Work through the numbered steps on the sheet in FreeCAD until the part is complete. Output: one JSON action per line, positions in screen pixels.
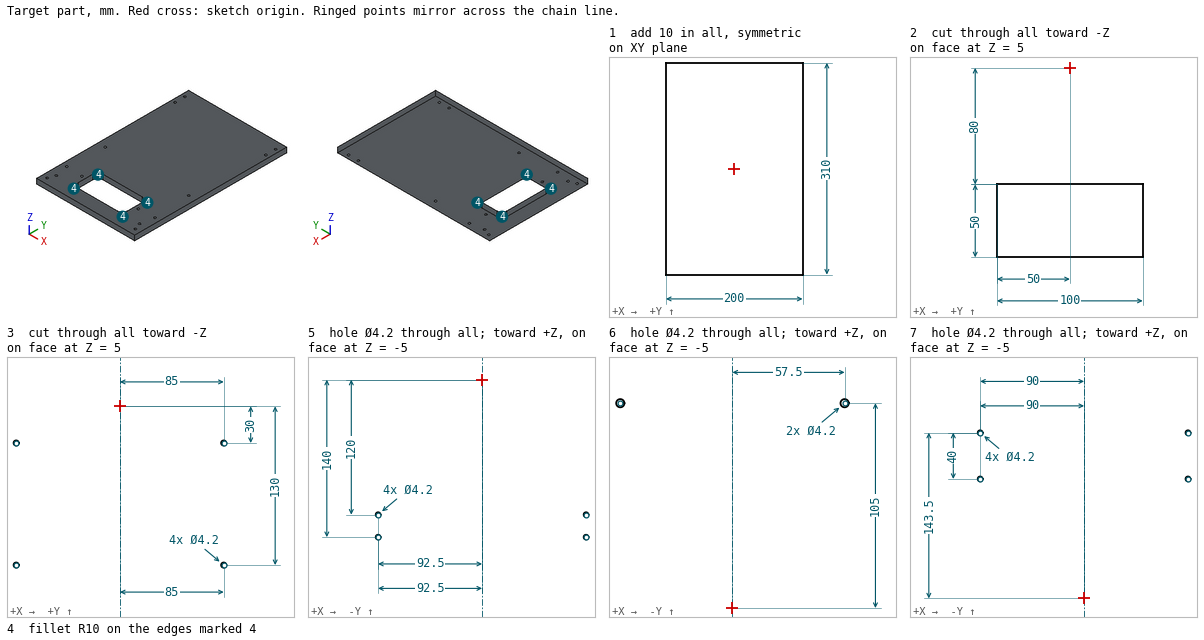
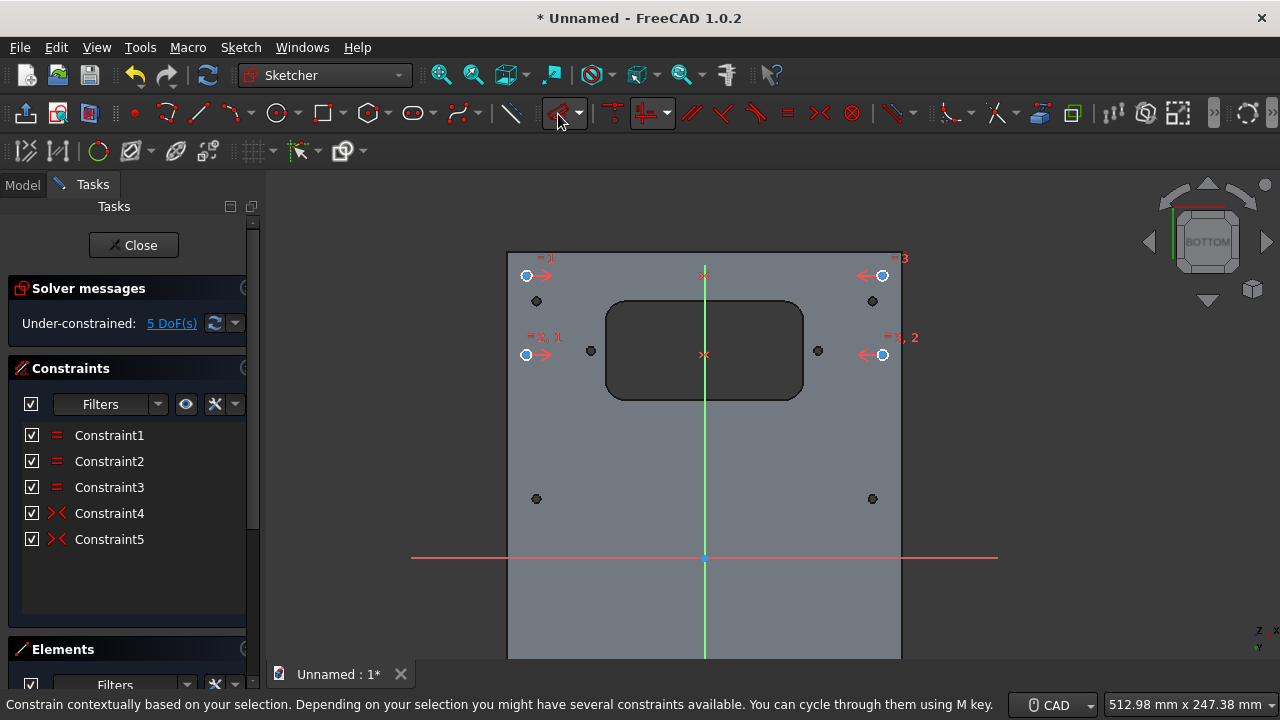
{"action": "scroll", "coordinate": [522, 276], "scroll_direction": "up", "scroll_amount": 8}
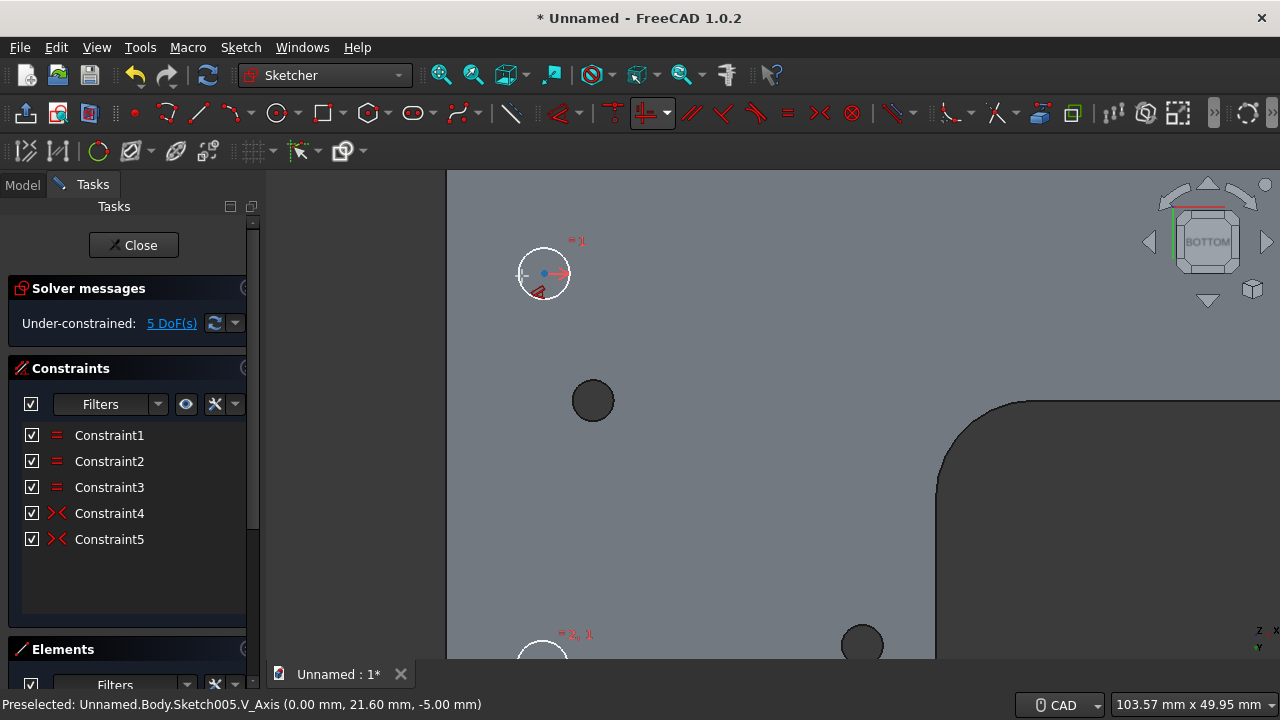
{"action": "left_click", "coordinate": [519, 273]}
{"action": "left_click", "coordinate": [487, 272]}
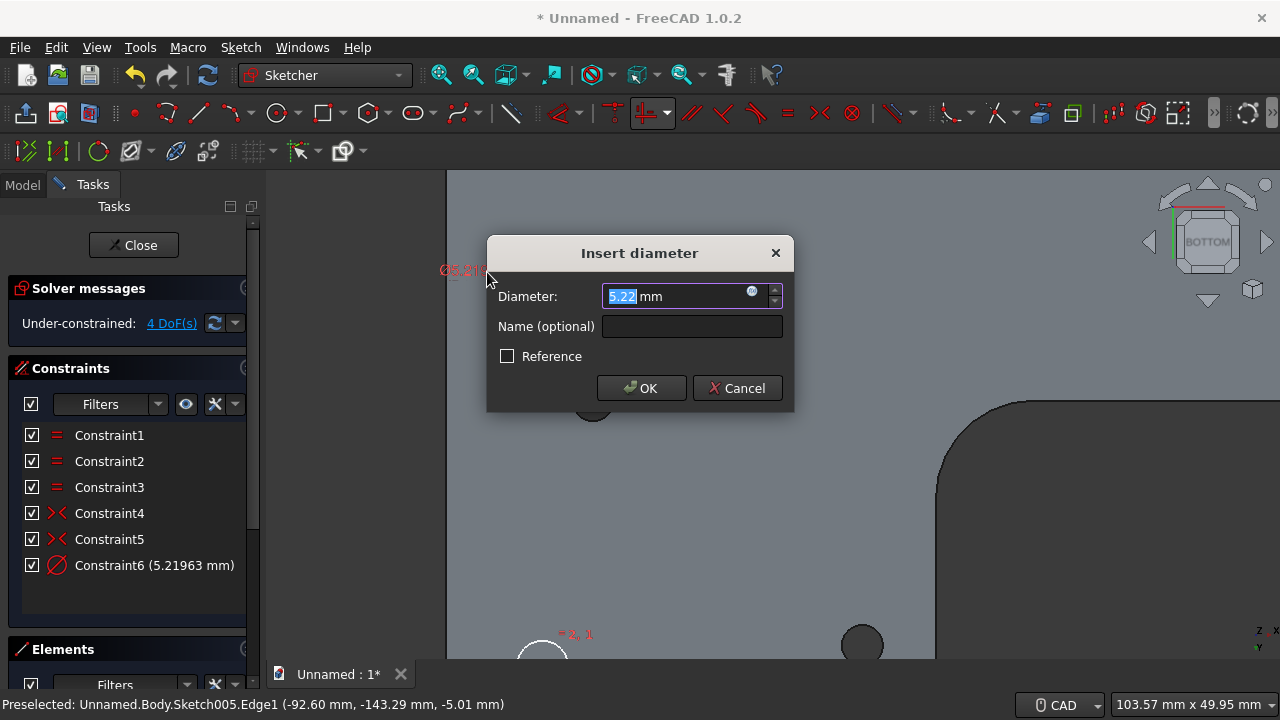
{"action": "type", "text": "4.2"}
{"action": "key", "text": "Return"}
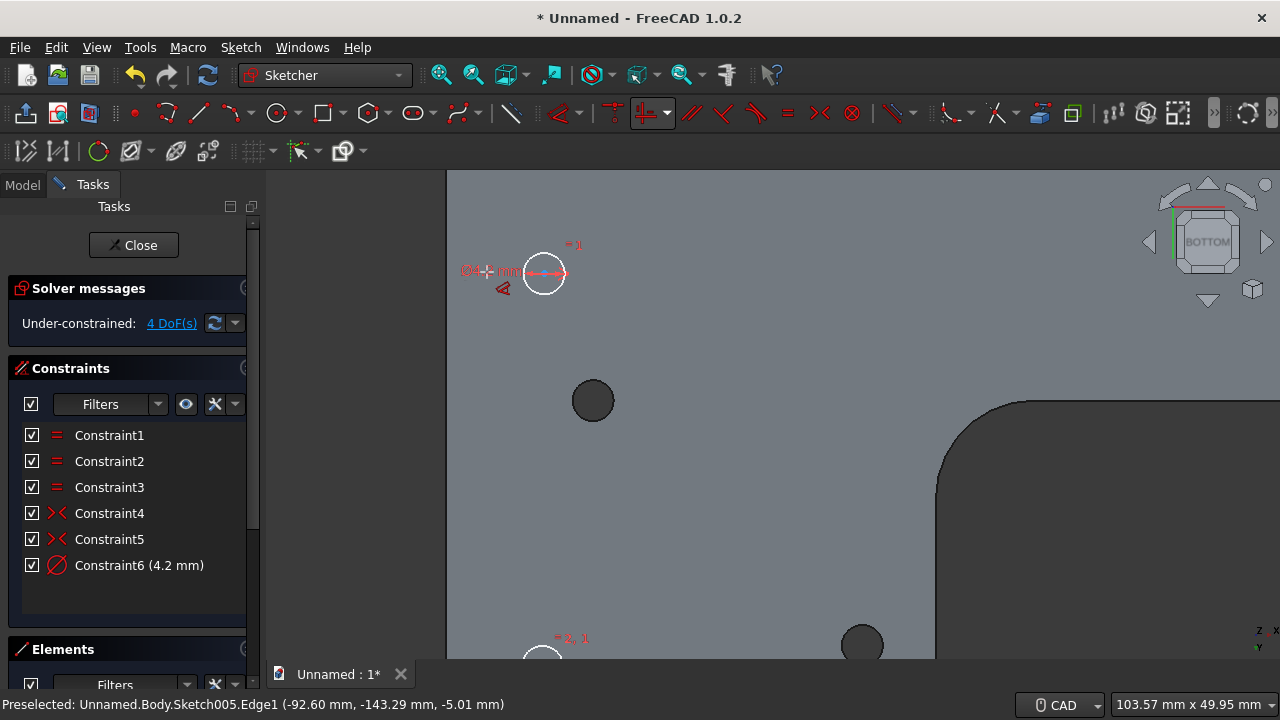
{"action": "scroll", "coordinate": [522, 276], "scroll_direction": "down", "scroll_amount": 8}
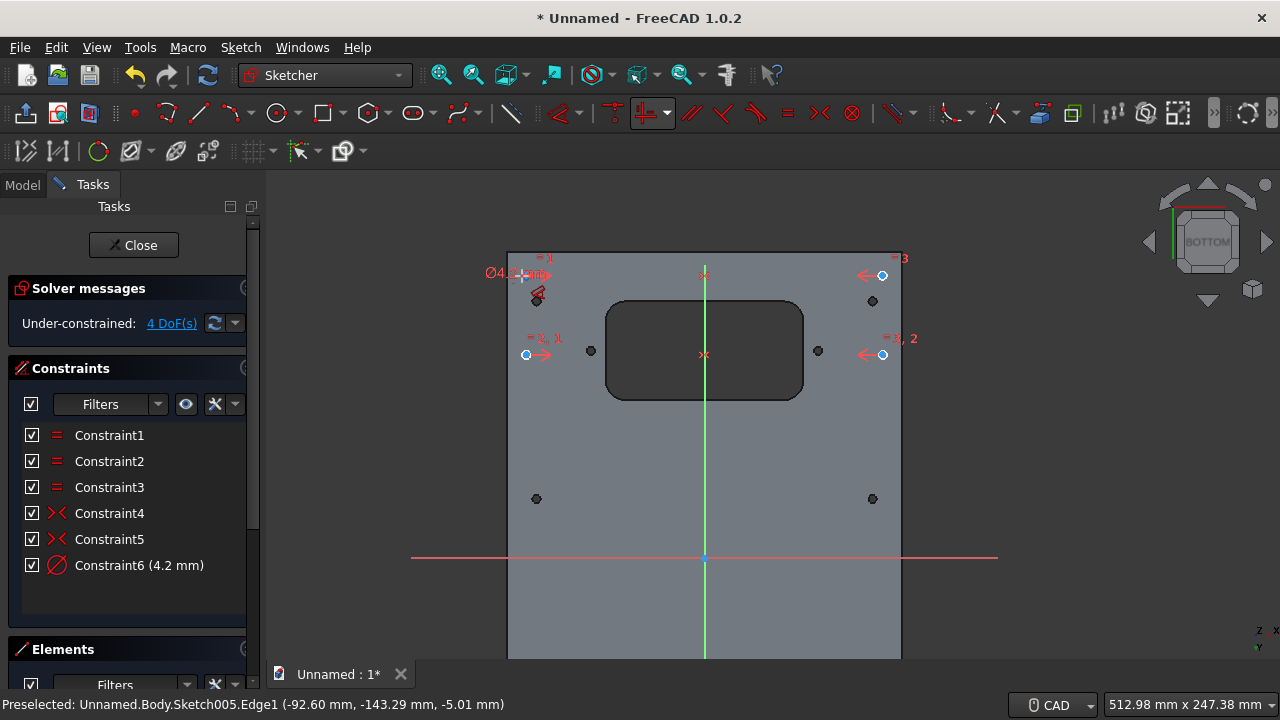
{"action": "left_click", "coordinate": [527, 276]}
{"action": "left_click", "coordinate": [616, 592]}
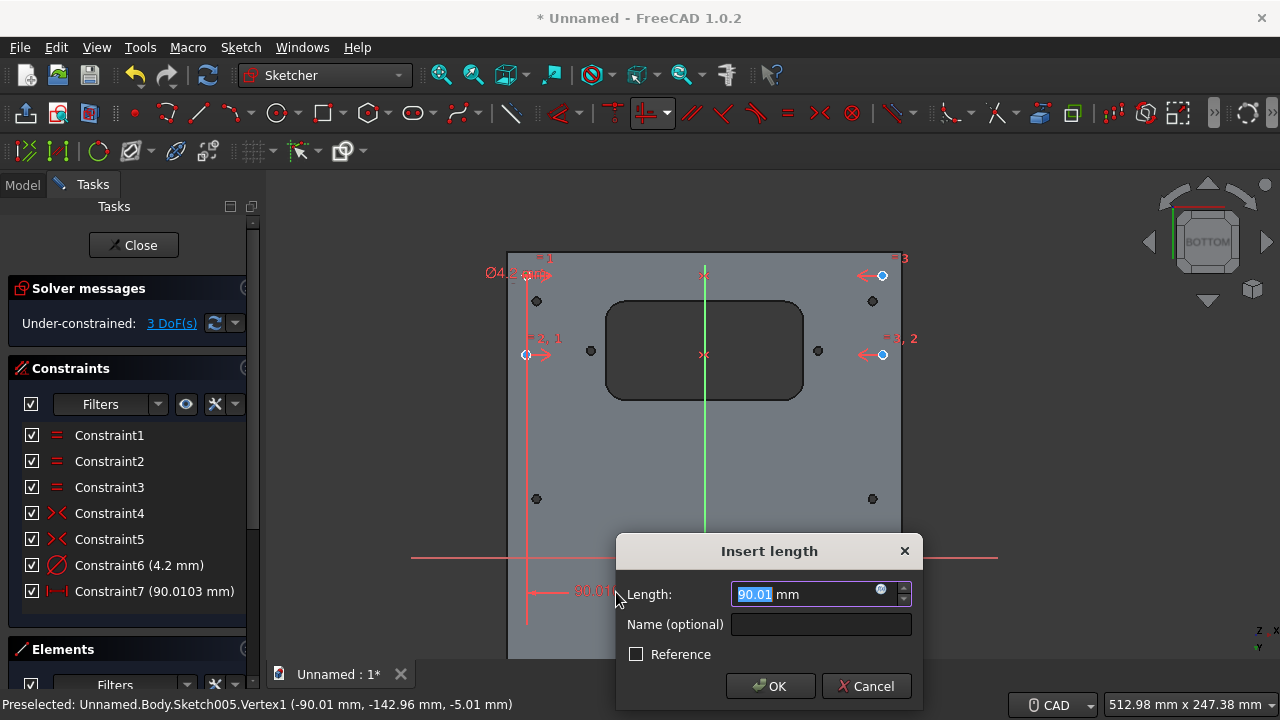
{"action": "type", "text": "90"}
{"action": "key", "text": "Return"}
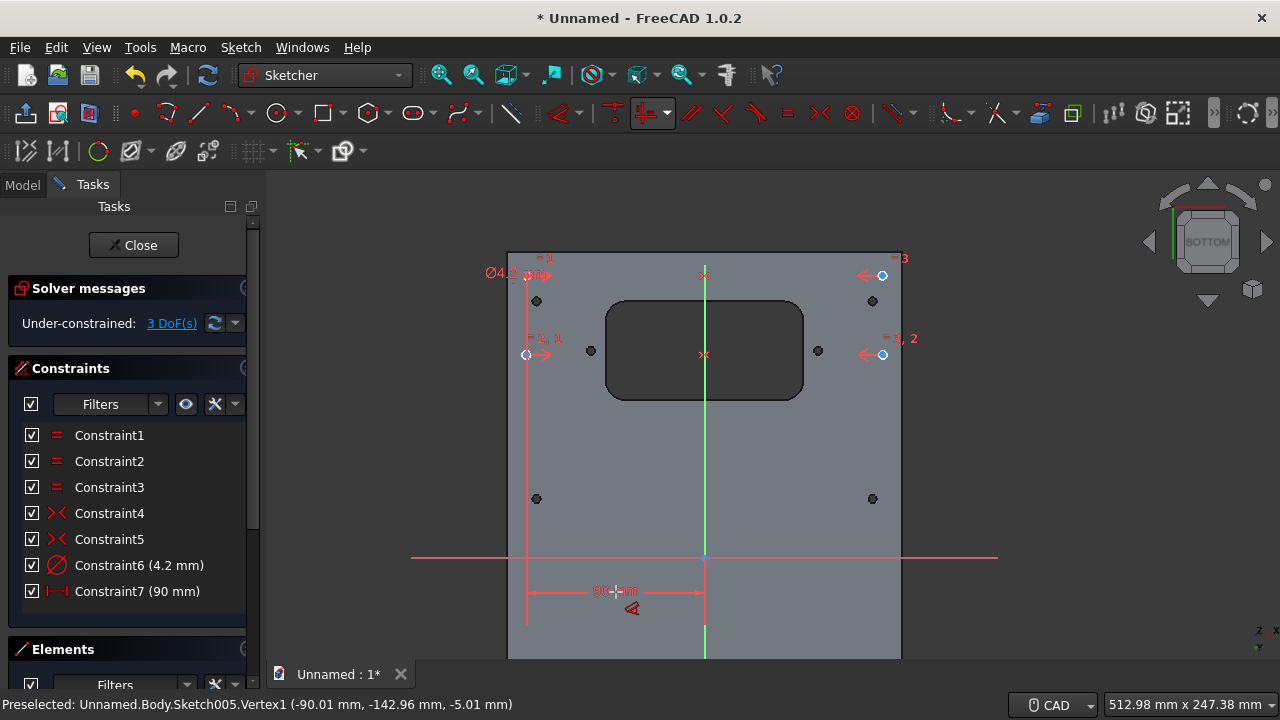
{"action": "left_click", "coordinate": [526, 355]}
{"action": "left_click", "coordinate": [615, 321]}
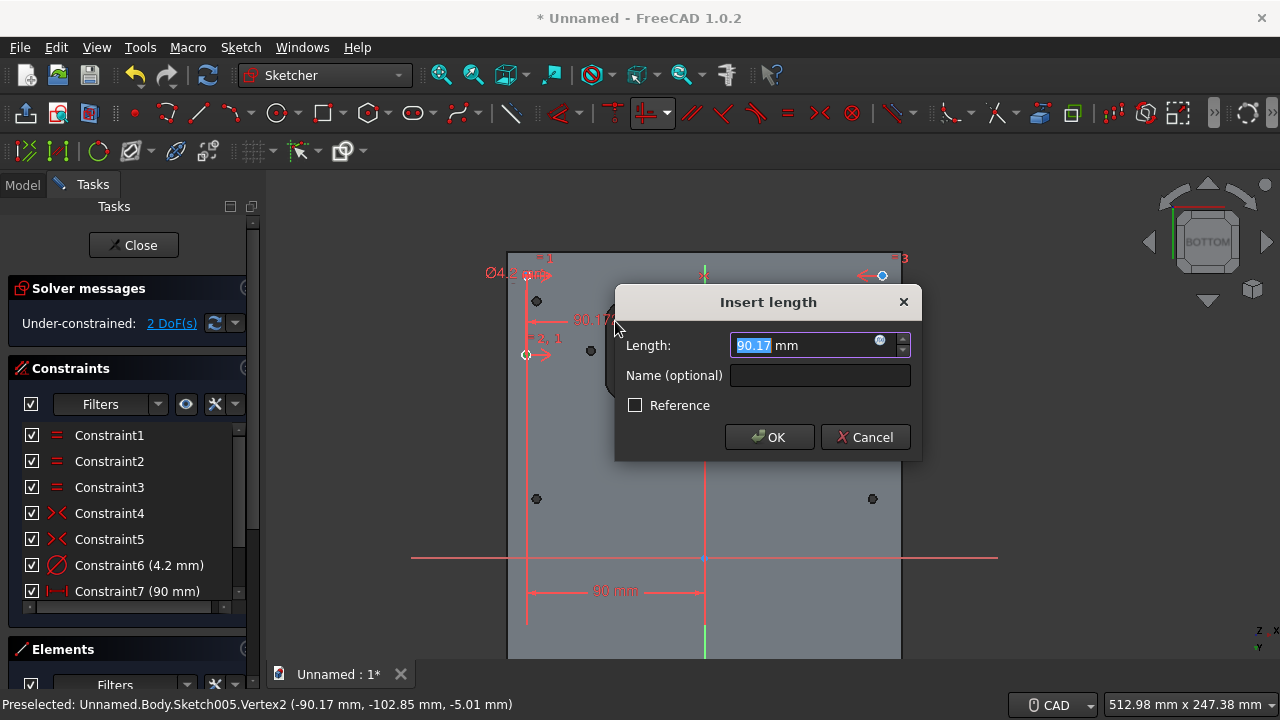
{"action": "type", "text": "90"}
{"action": "key", "text": "Return"}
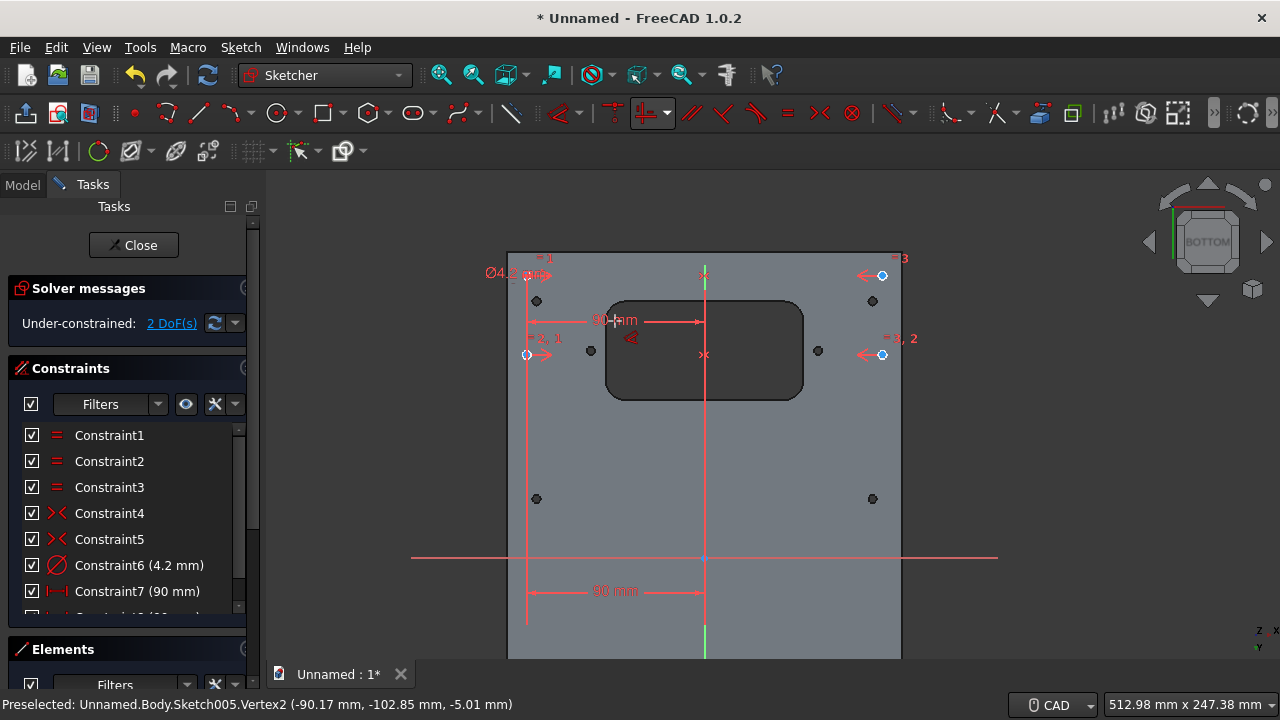
{"action": "left_click", "coordinate": [527, 276]}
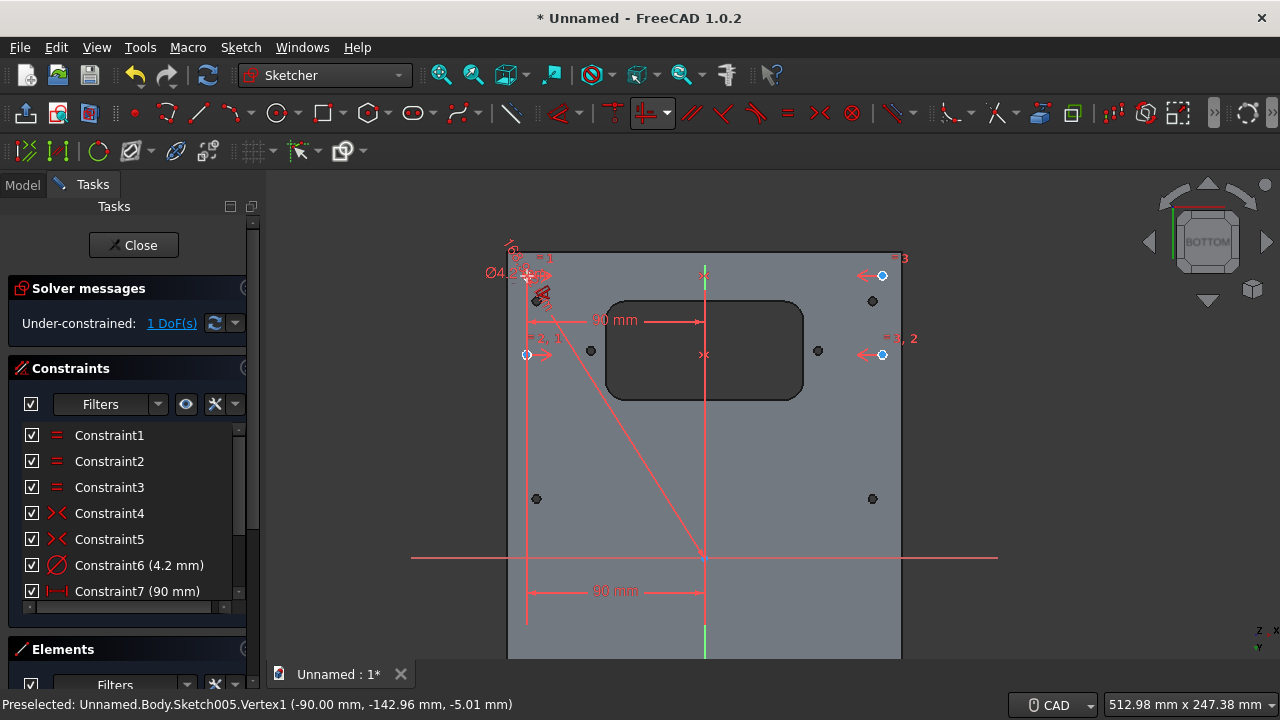
{"action": "left_click", "coordinate": [527, 355]}
{"action": "left_click", "coordinate": [493, 315]}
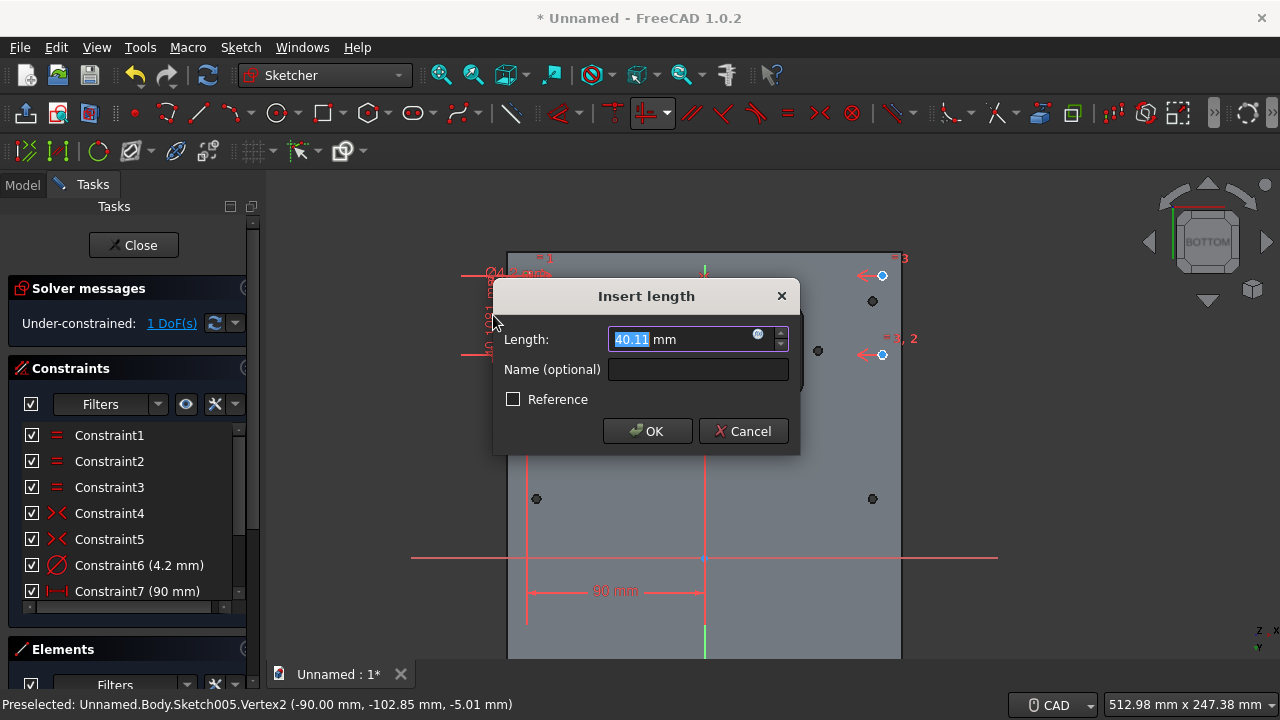
{"action": "type", "text": "40"}
{"action": "key", "text": "Return"}